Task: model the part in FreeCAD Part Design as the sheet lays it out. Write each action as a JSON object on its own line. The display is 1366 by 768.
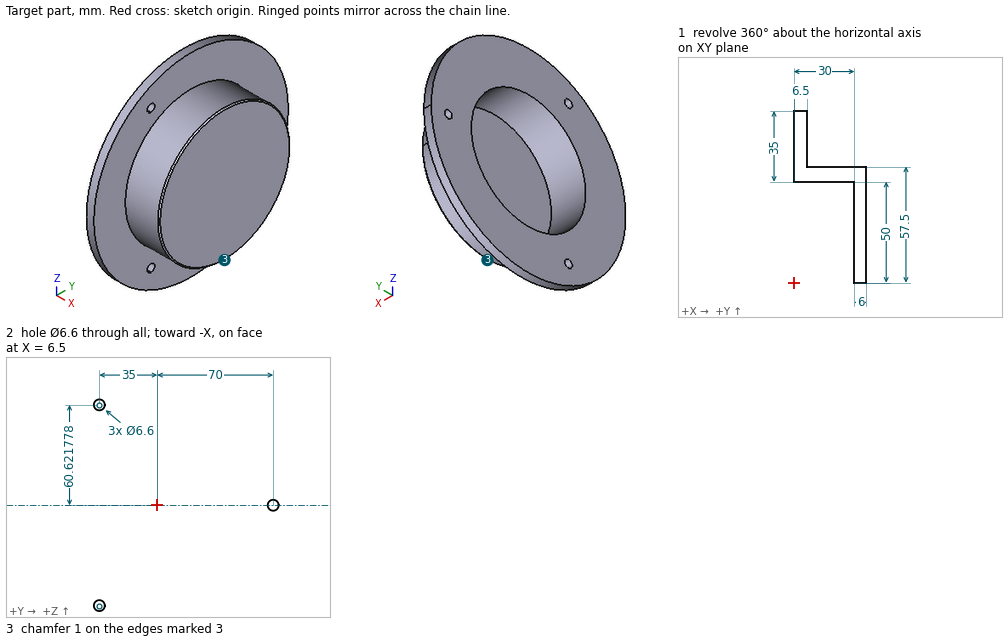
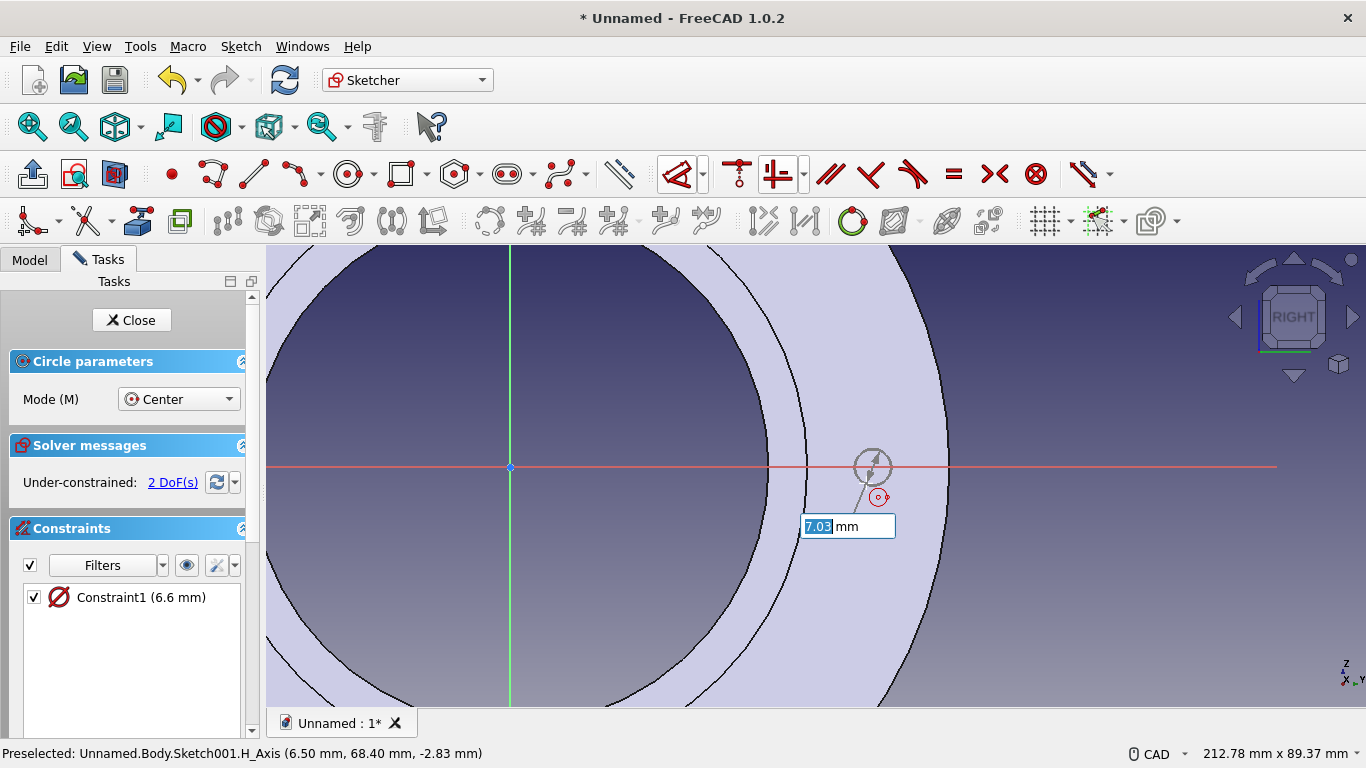
{"action": "type", "text": "6.6"}
{"action": "key", "text": "Return"}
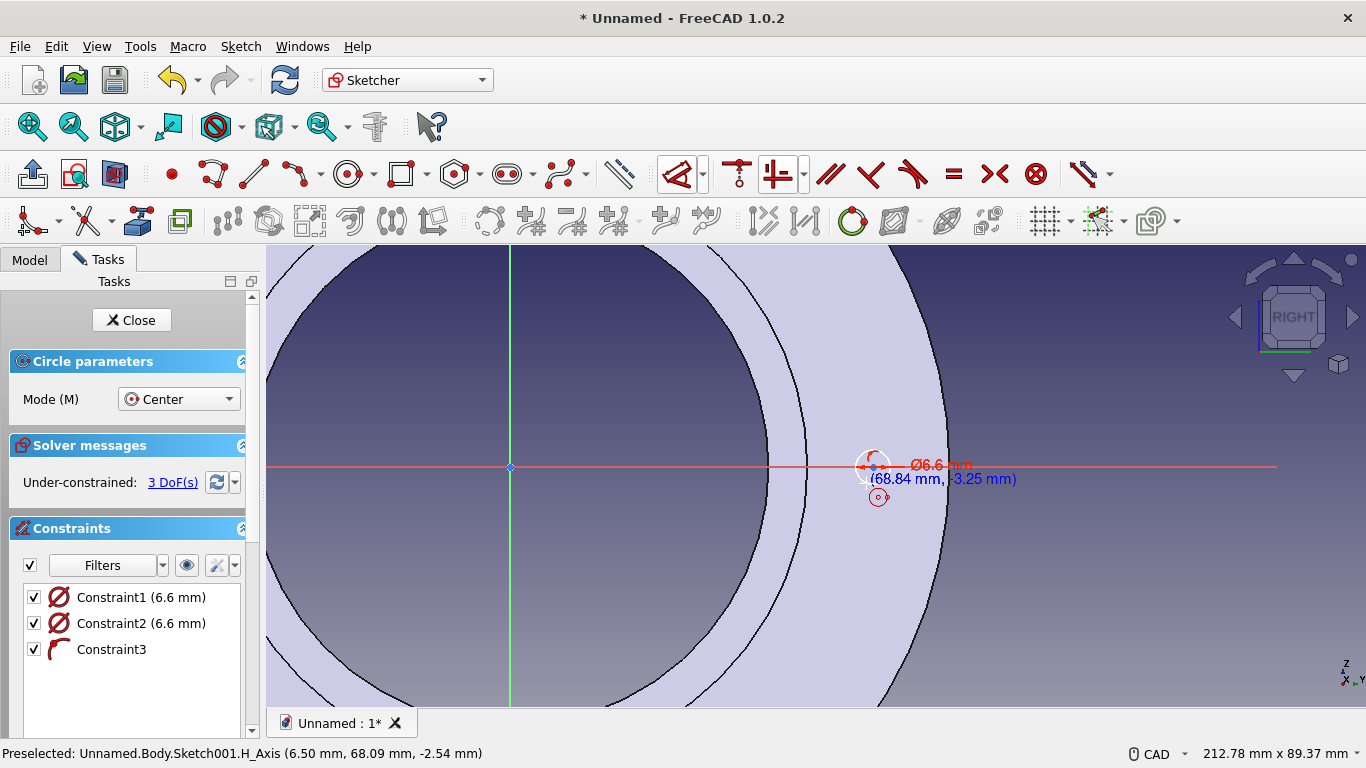
{"action": "scroll", "coordinate": [867, 483], "scroll_direction": "down", "scroll_amount": 4}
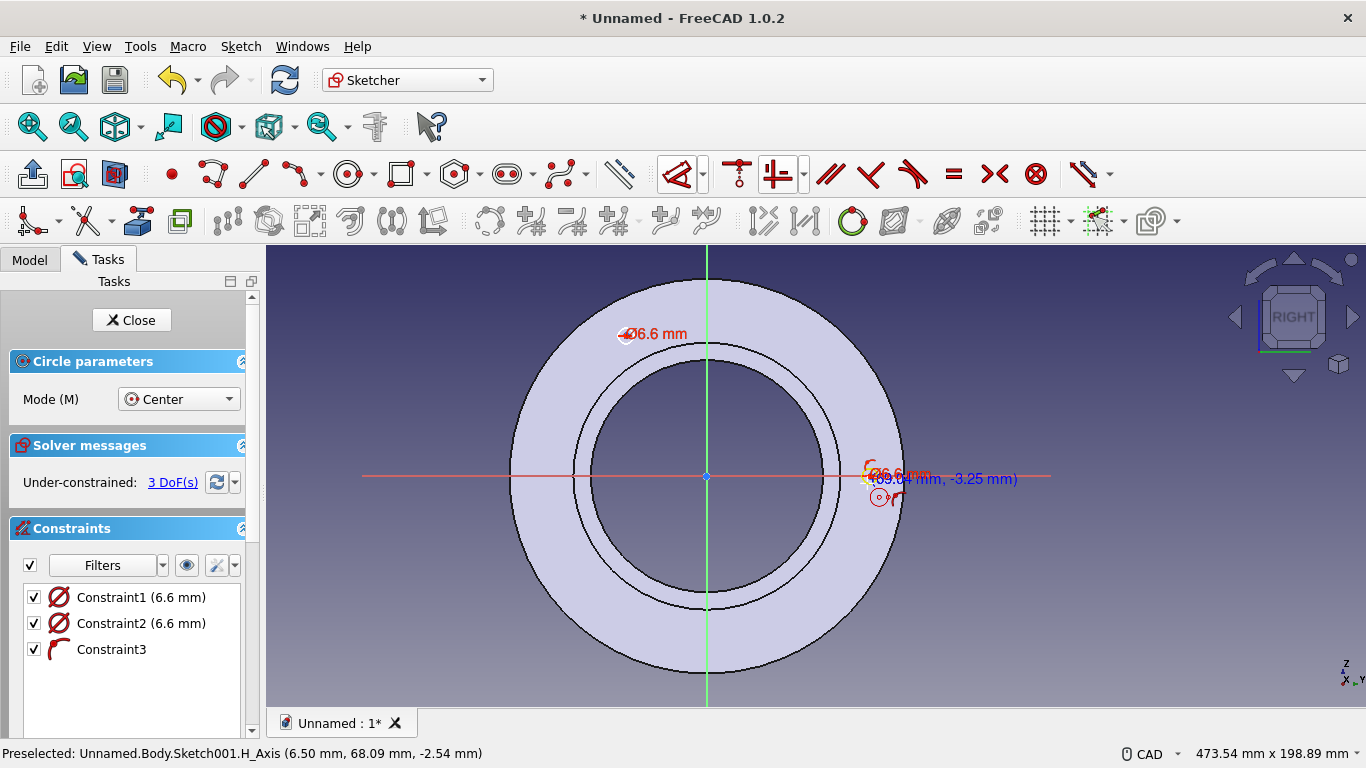
{"action": "scroll", "coordinate": [626, 617], "scroll_direction": "up", "scroll_amount": 6}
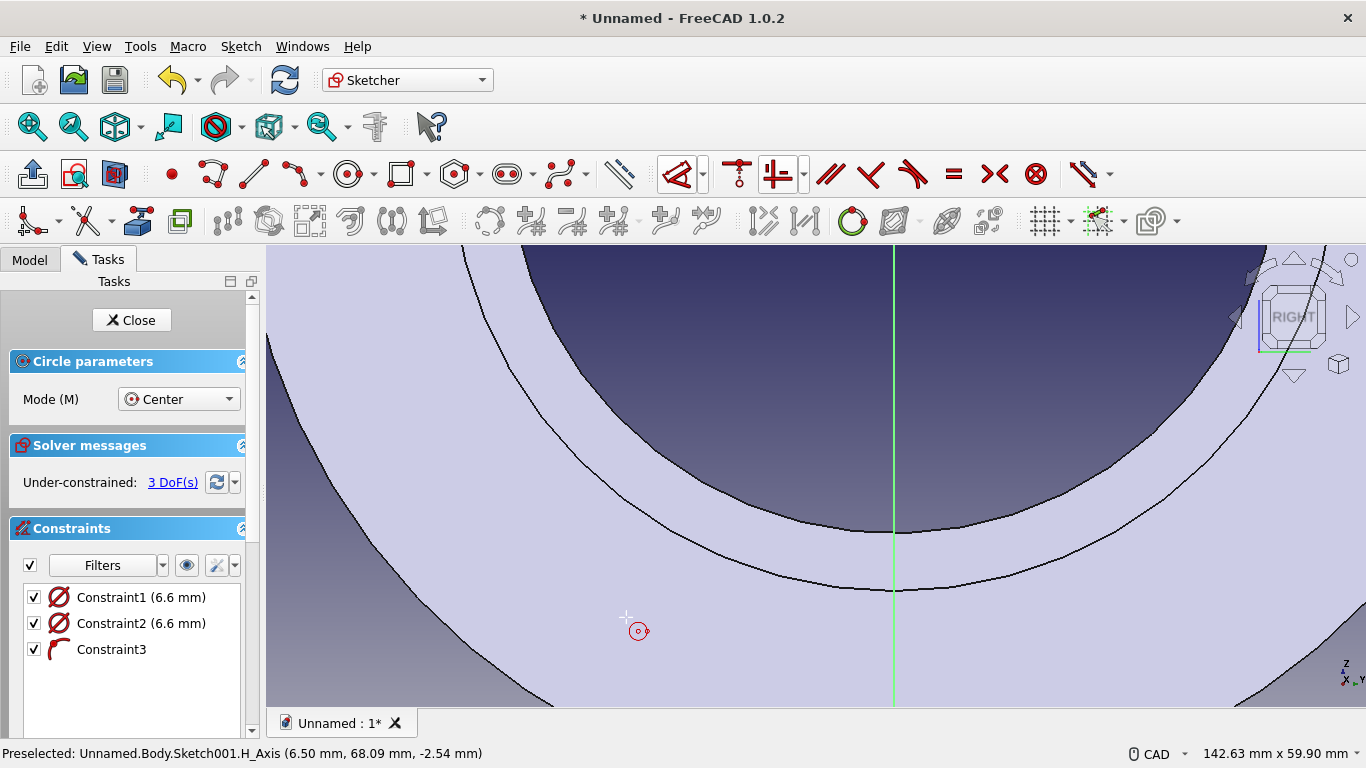
{"action": "scroll", "coordinate": [626, 618], "scroll_direction": "down", "scroll_amount": 6}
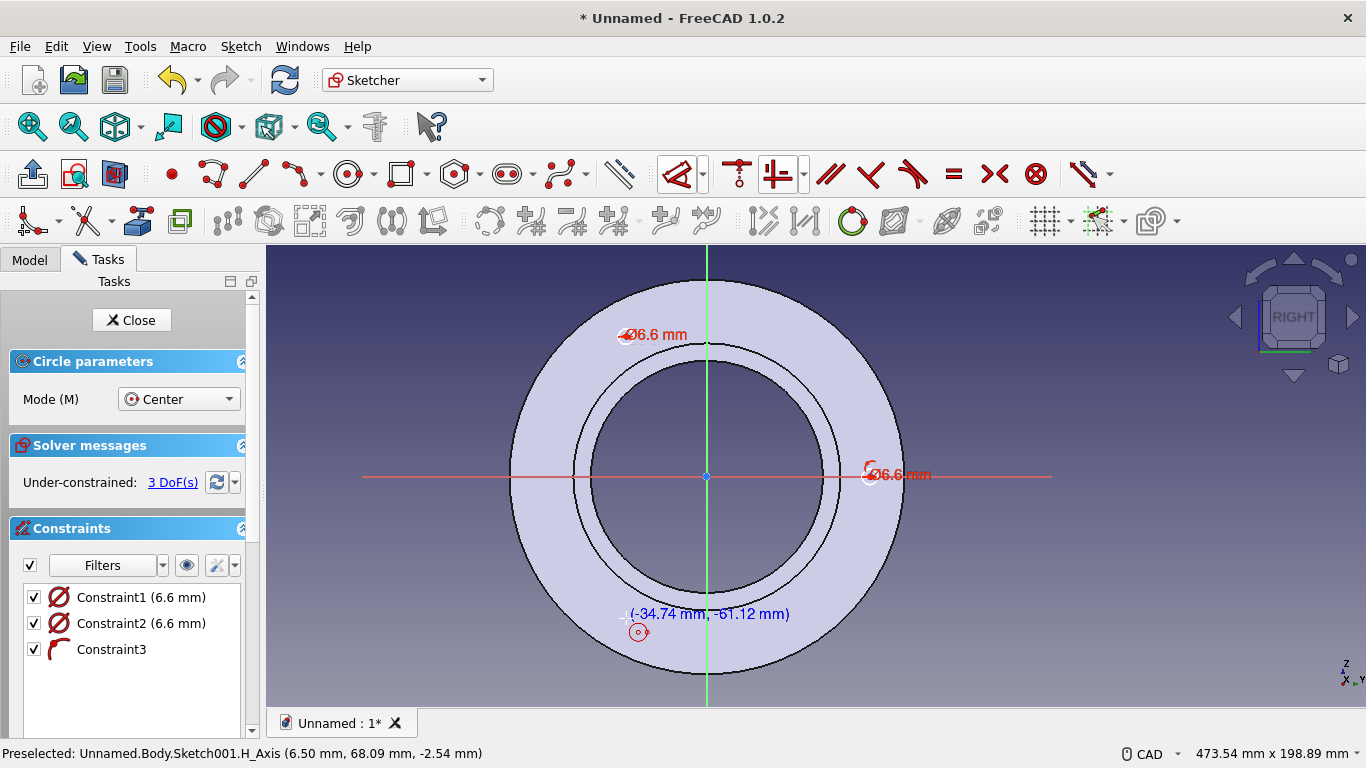
{"action": "left_click", "coordinate": [626, 618]}
{"action": "mouse_move", "coordinate": [631, 612]}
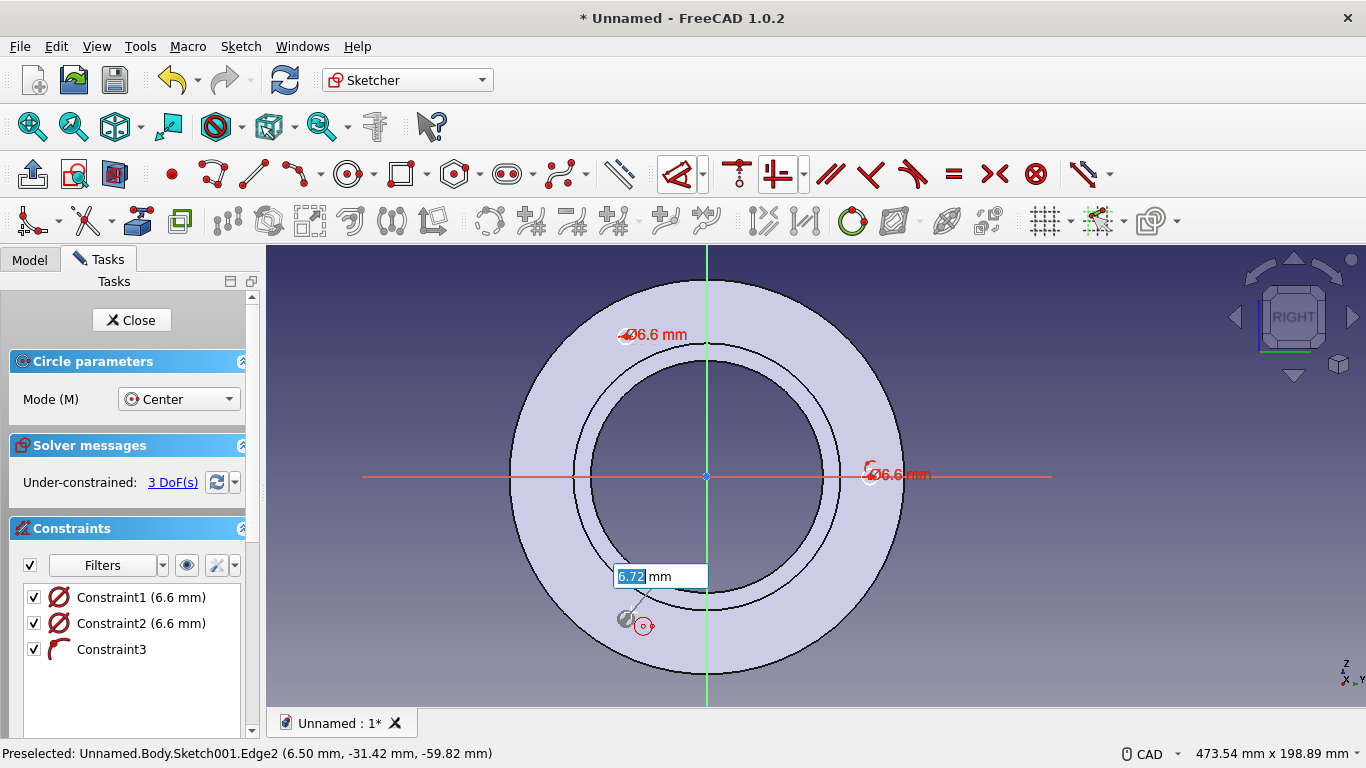
{"action": "type", "text": "6.6"}
{"action": "key", "text": "Return"}
{"action": "key", "text": "Escape"}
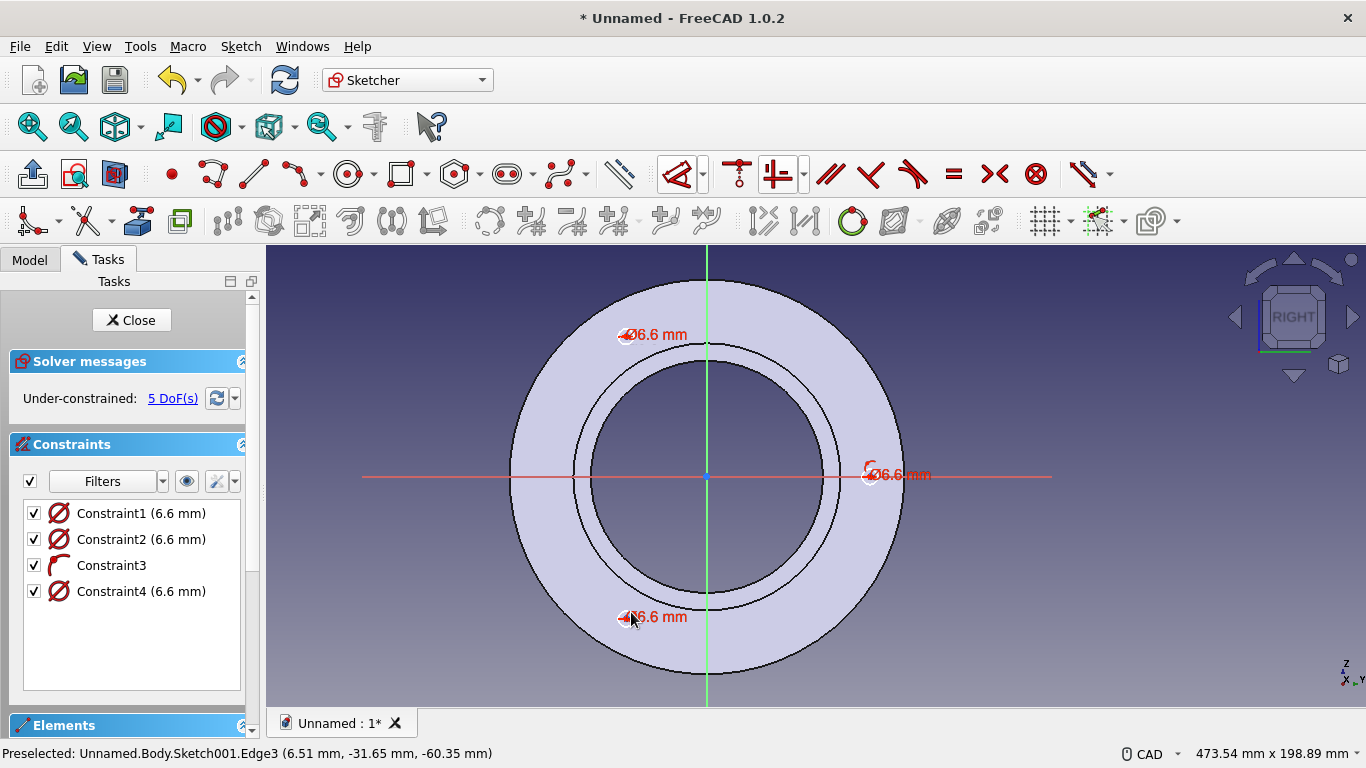
{"action": "left_click", "coordinate": [626, 337]}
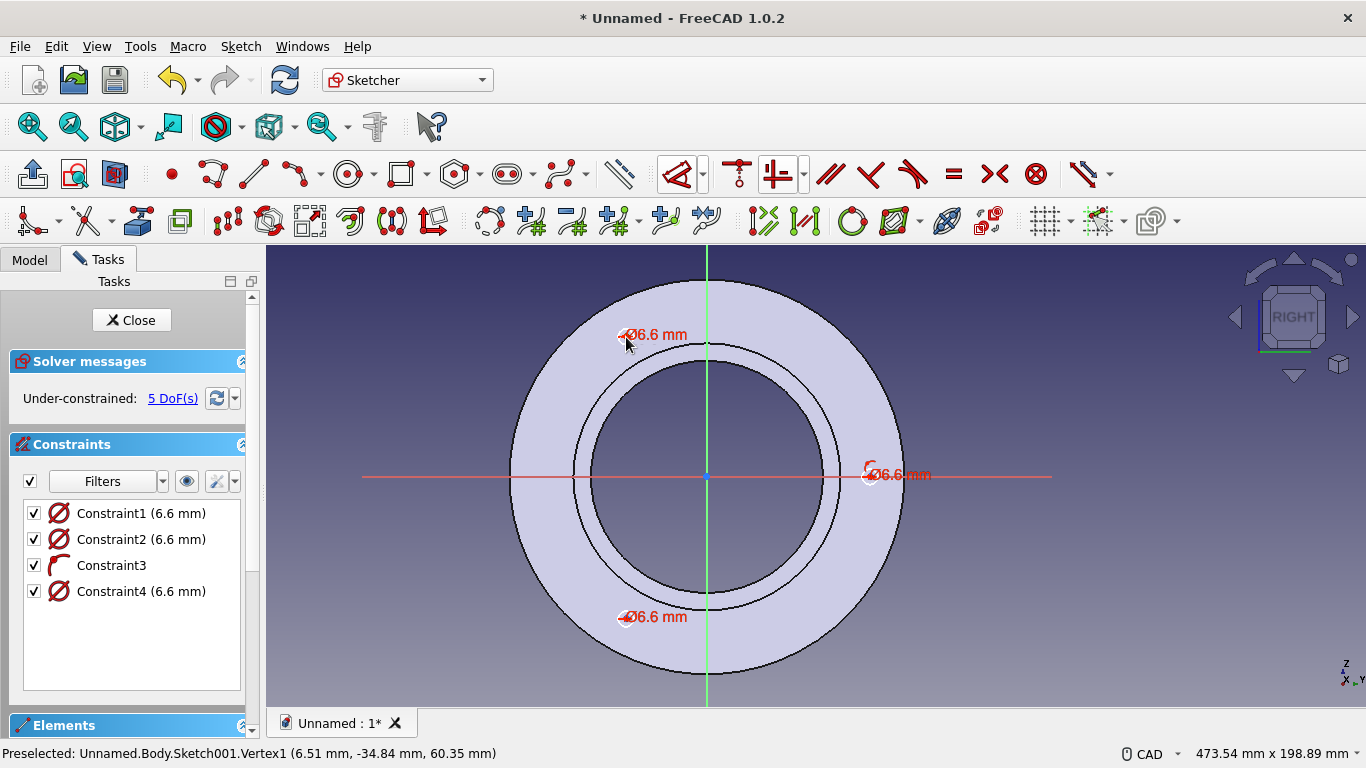
{"action": "left_click", "coordinate": [626, 619]}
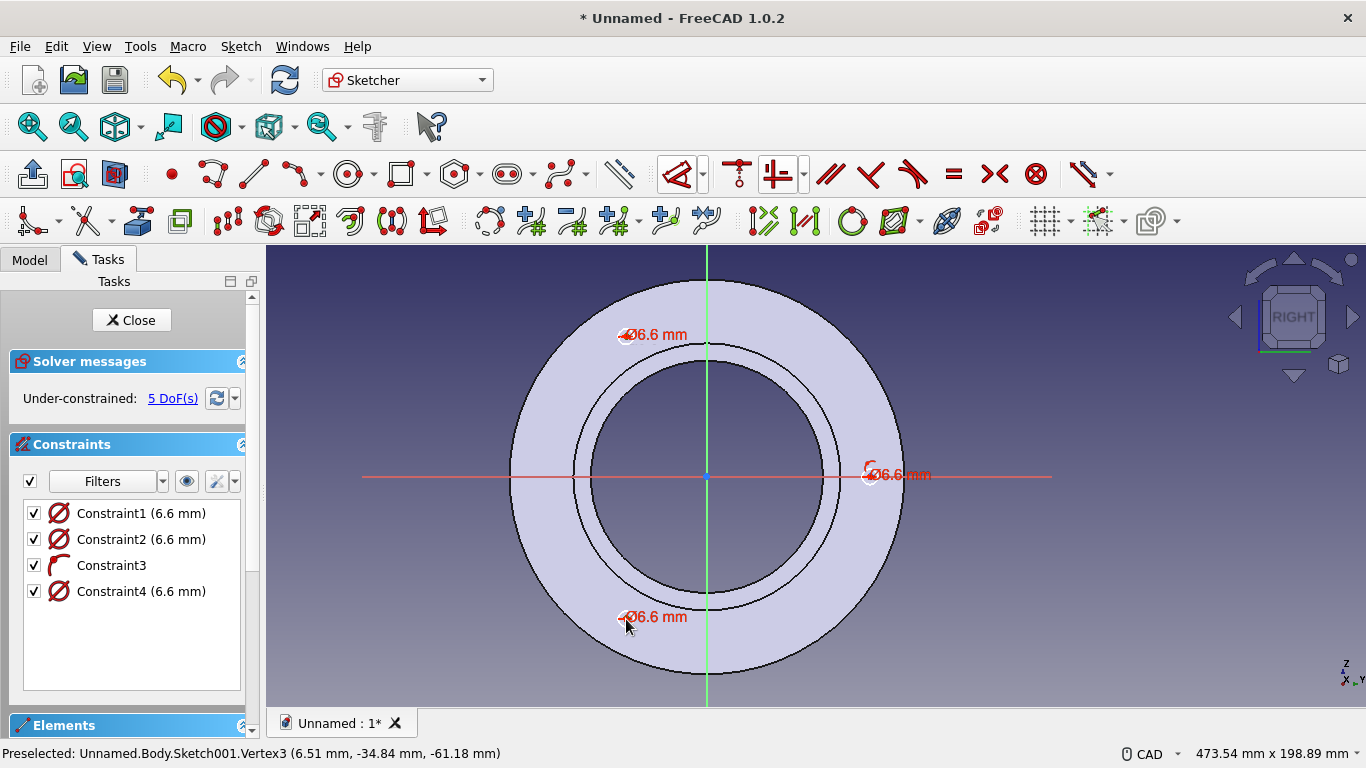
{"action": "left_click", "coordinate": [359, 477]}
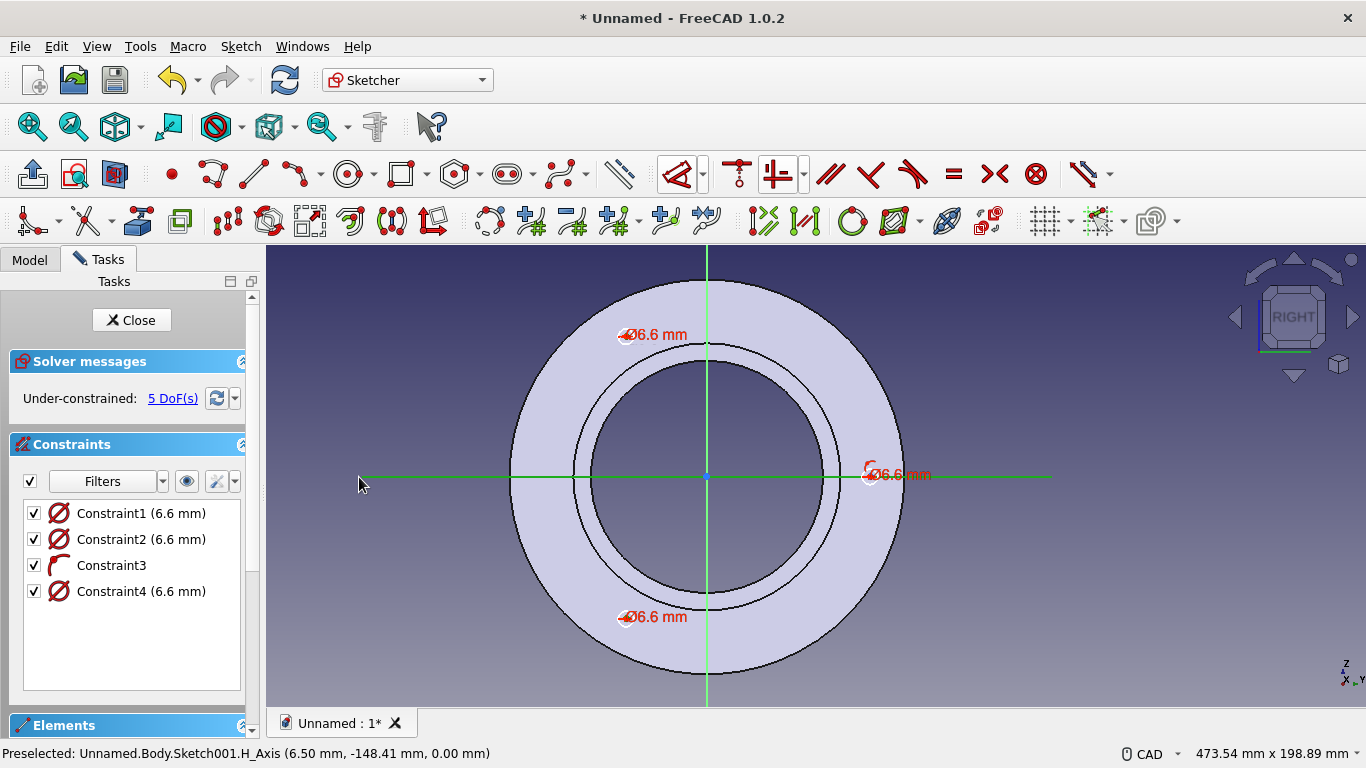
{"action": "left_click", "coordinate": [995, 174]}